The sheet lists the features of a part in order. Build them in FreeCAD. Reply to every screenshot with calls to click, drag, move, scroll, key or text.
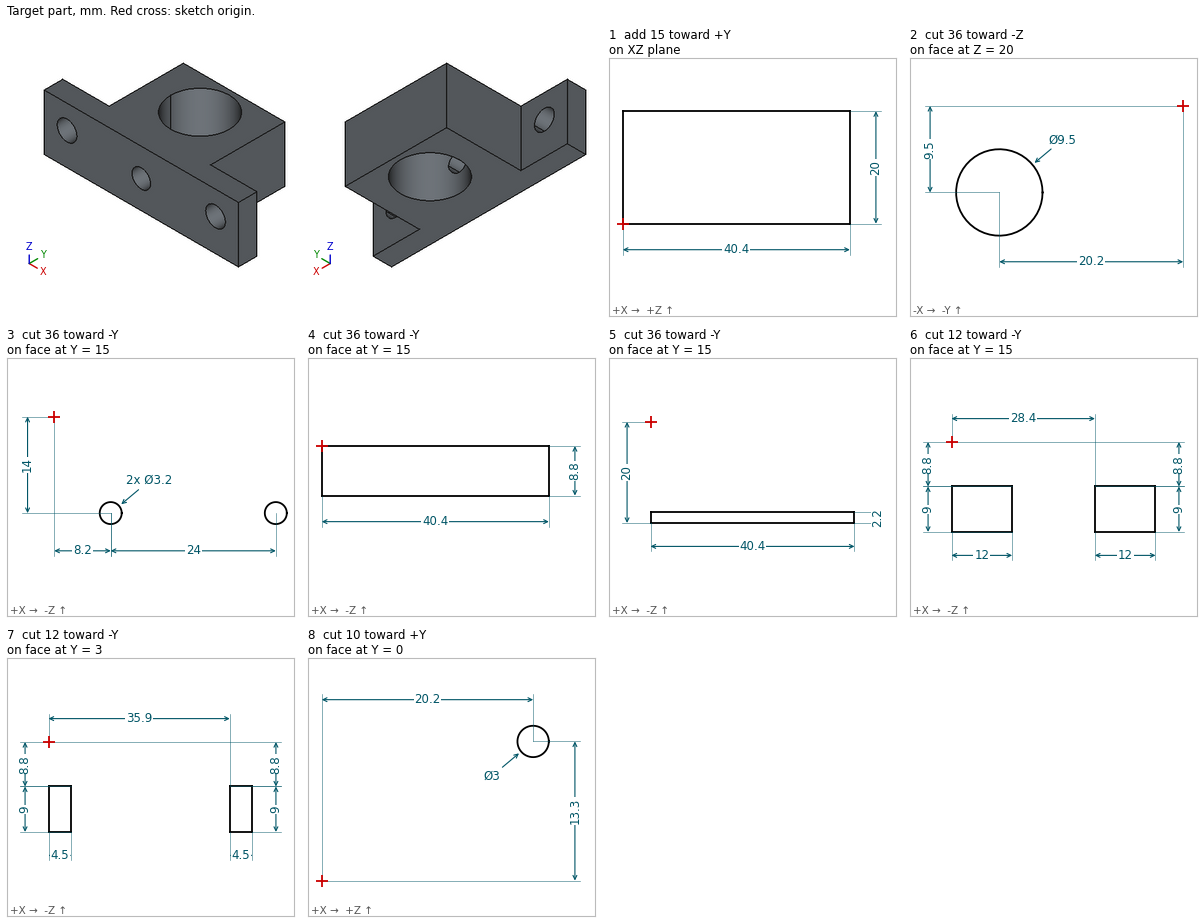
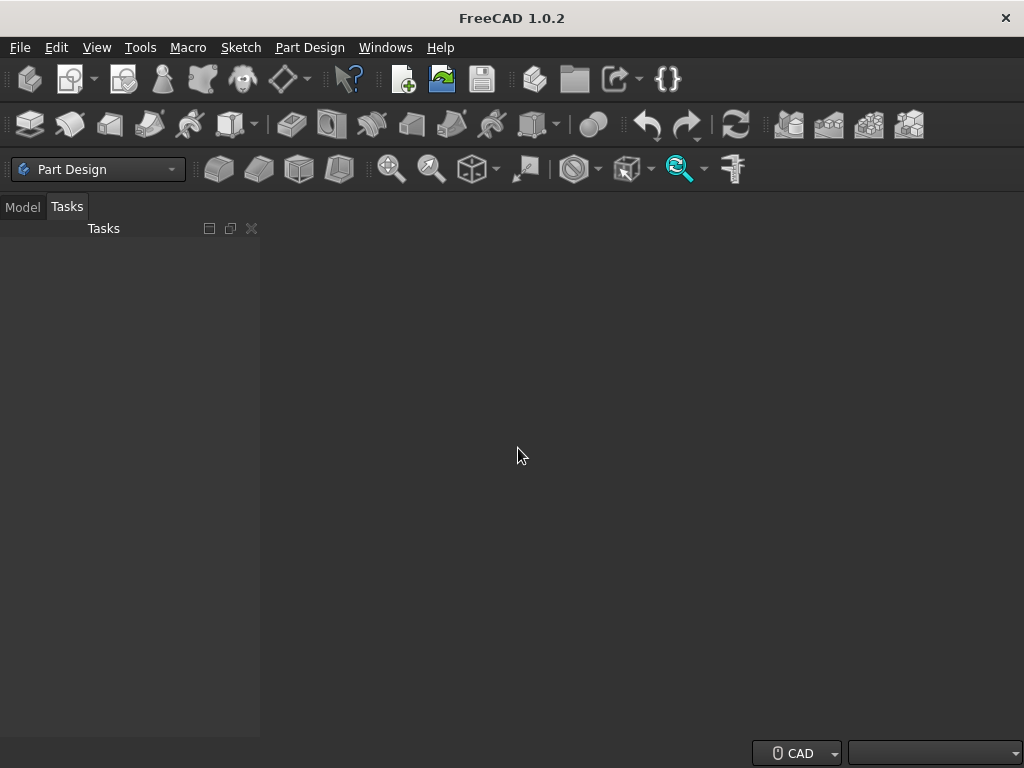
key(ctrl+n)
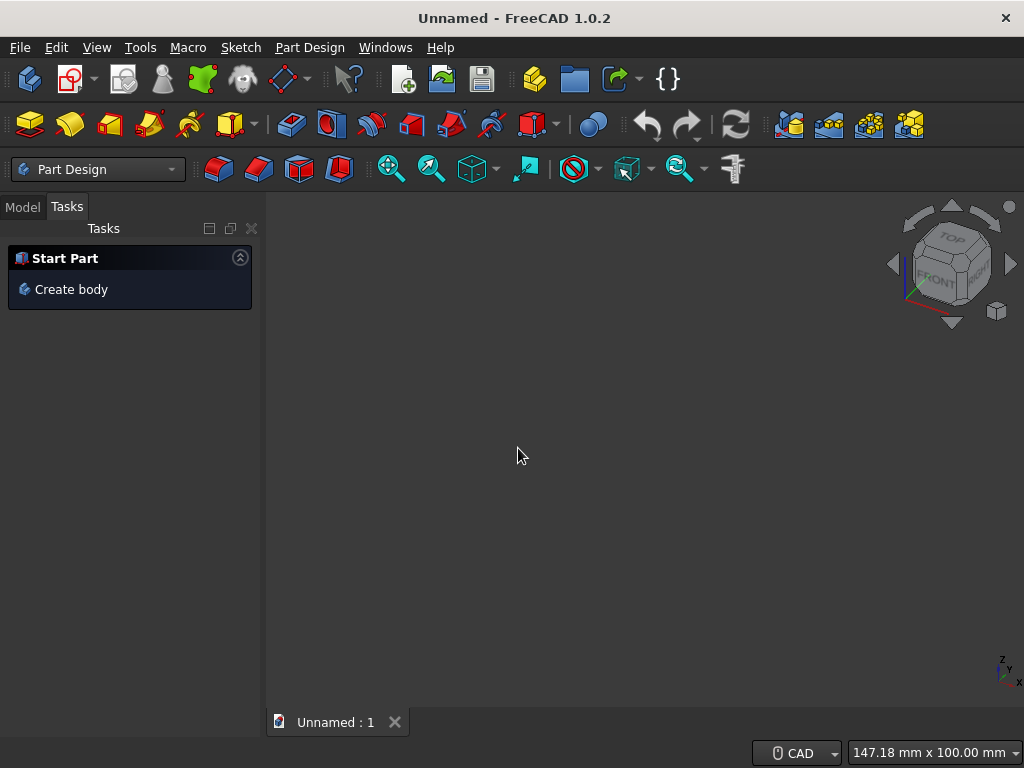
click(70, 80)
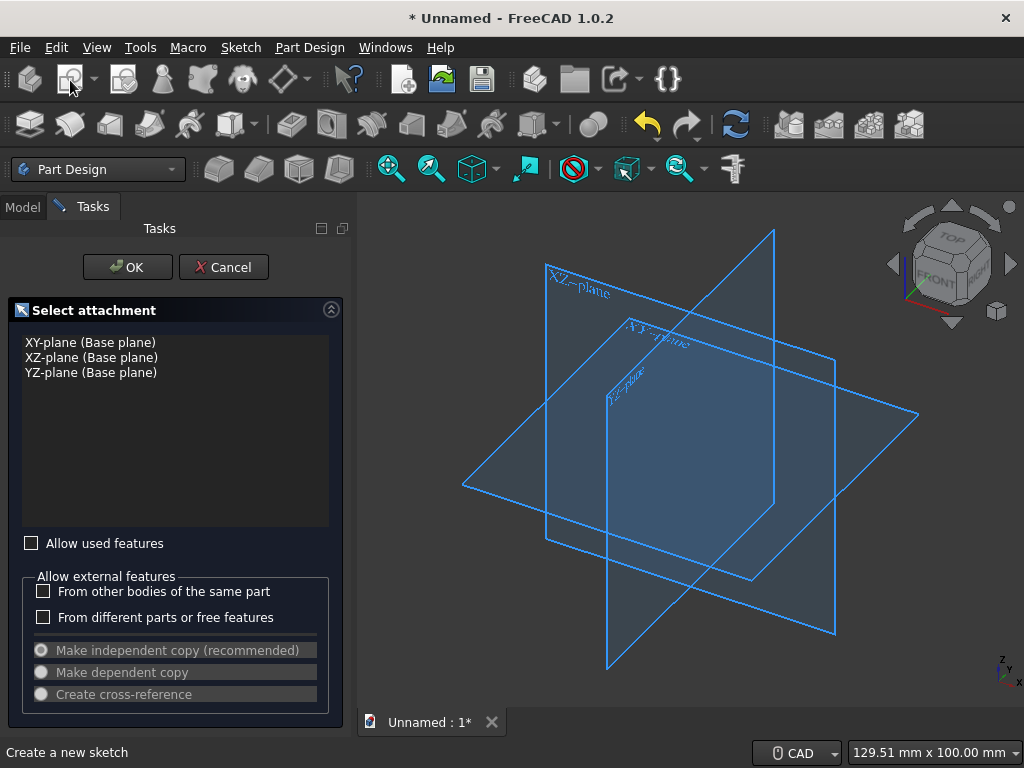
click(82, 358)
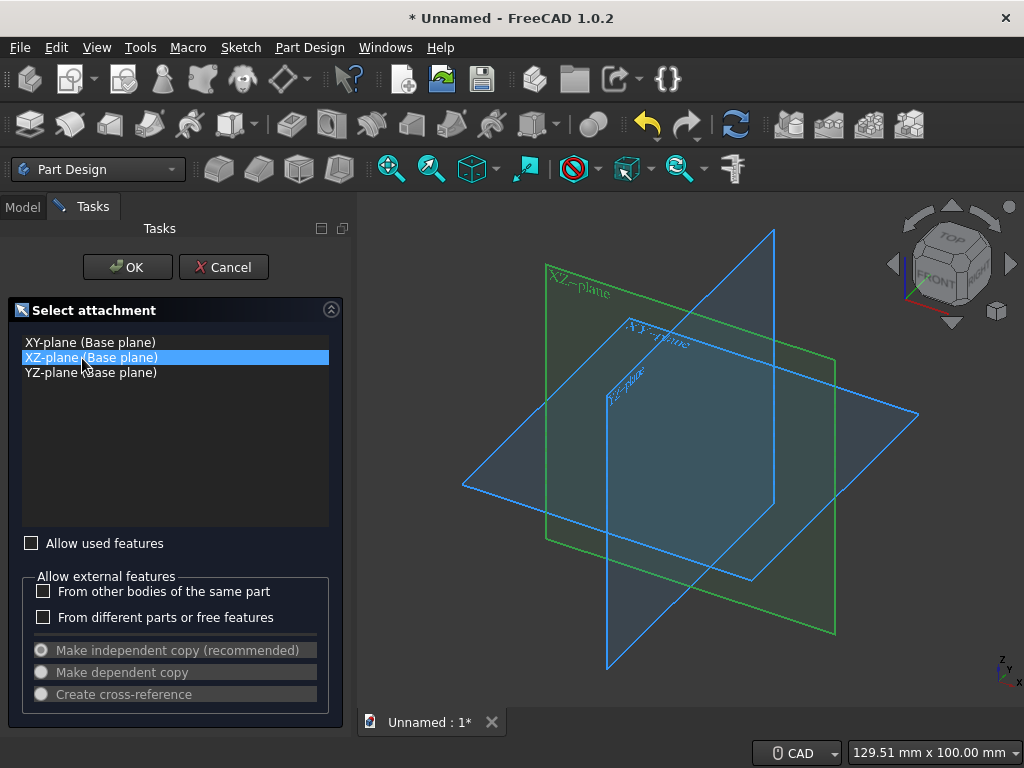
click(128, 267)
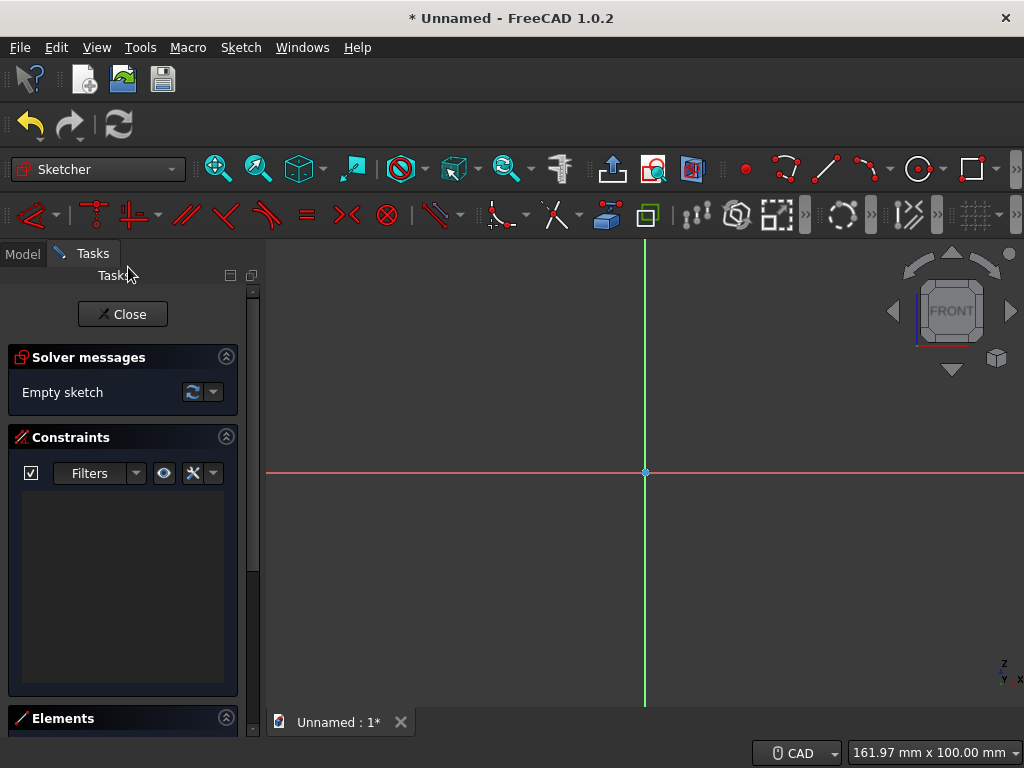
scroll(859, 388, up, 4)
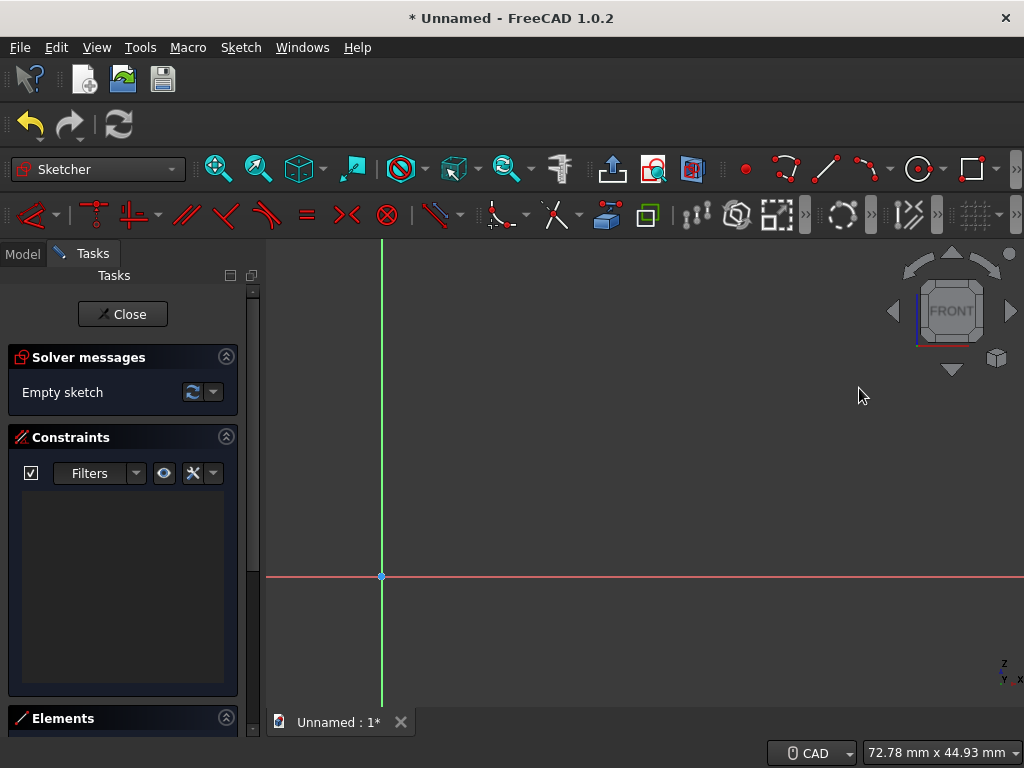
key(g)
key(r)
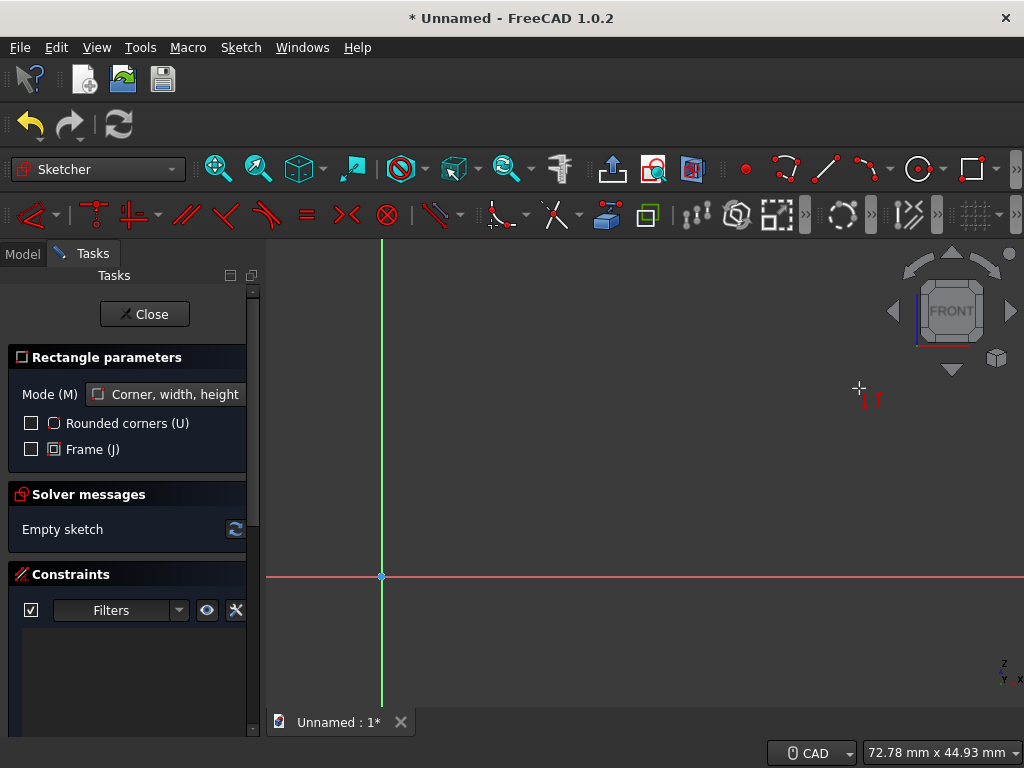
click(382, 577)
move(803, 368)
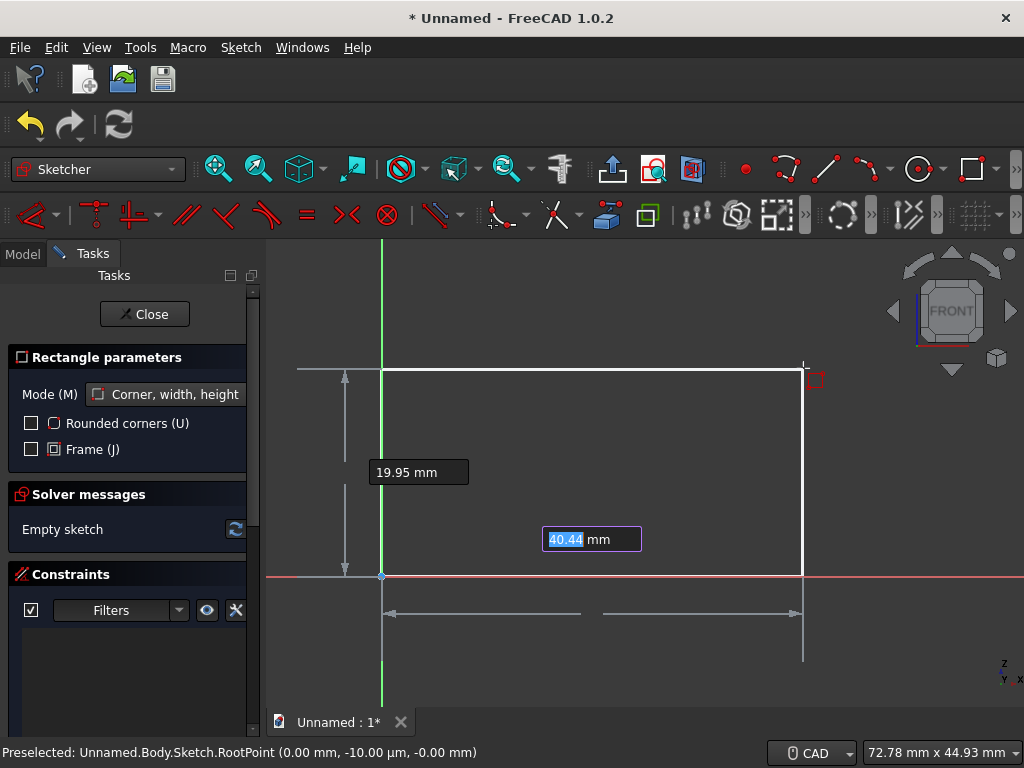
text(40.4)
key(Tab)
text(20)
key(Return)
key(Escape)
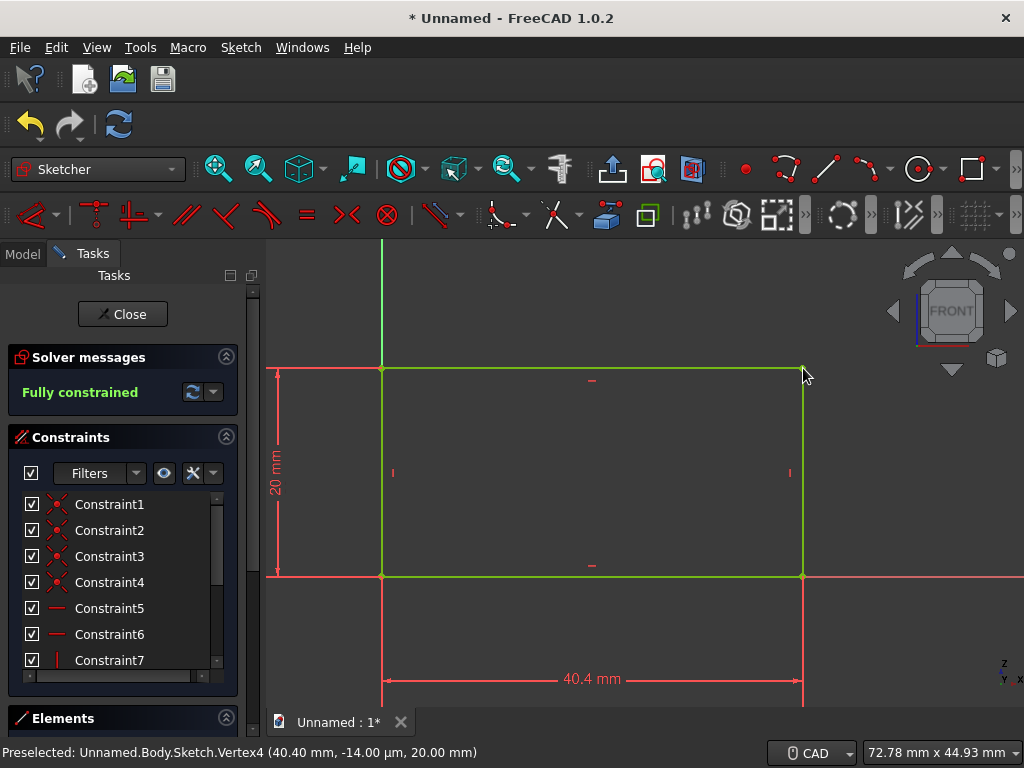
click(123, 314)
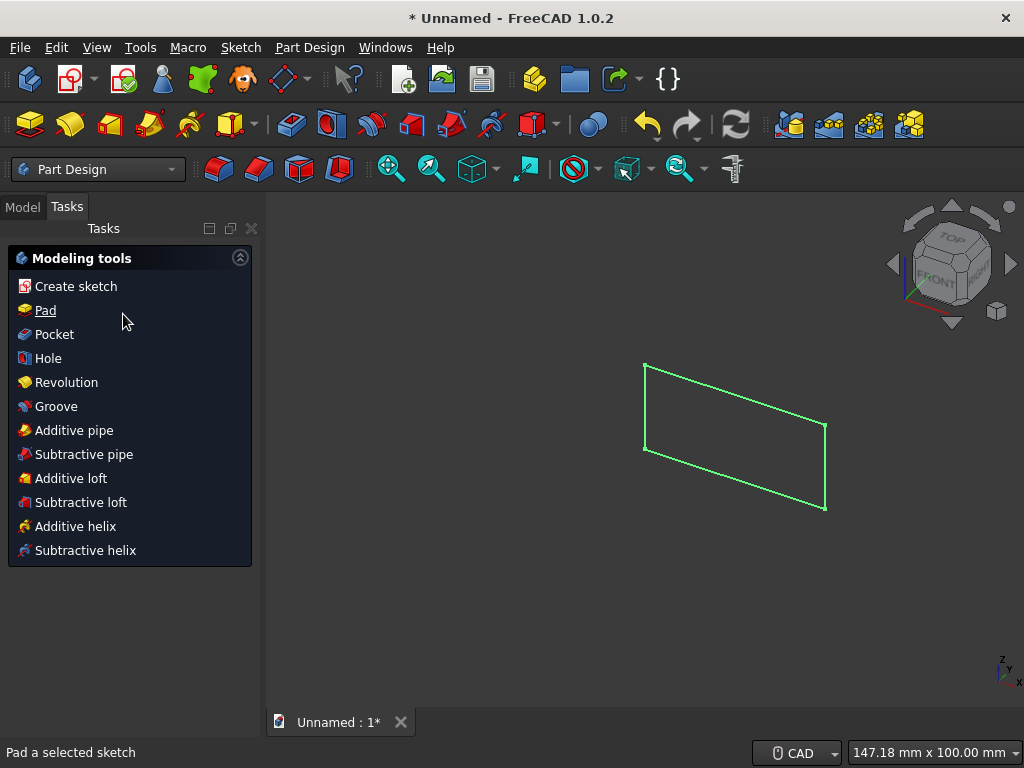
click(30, 124)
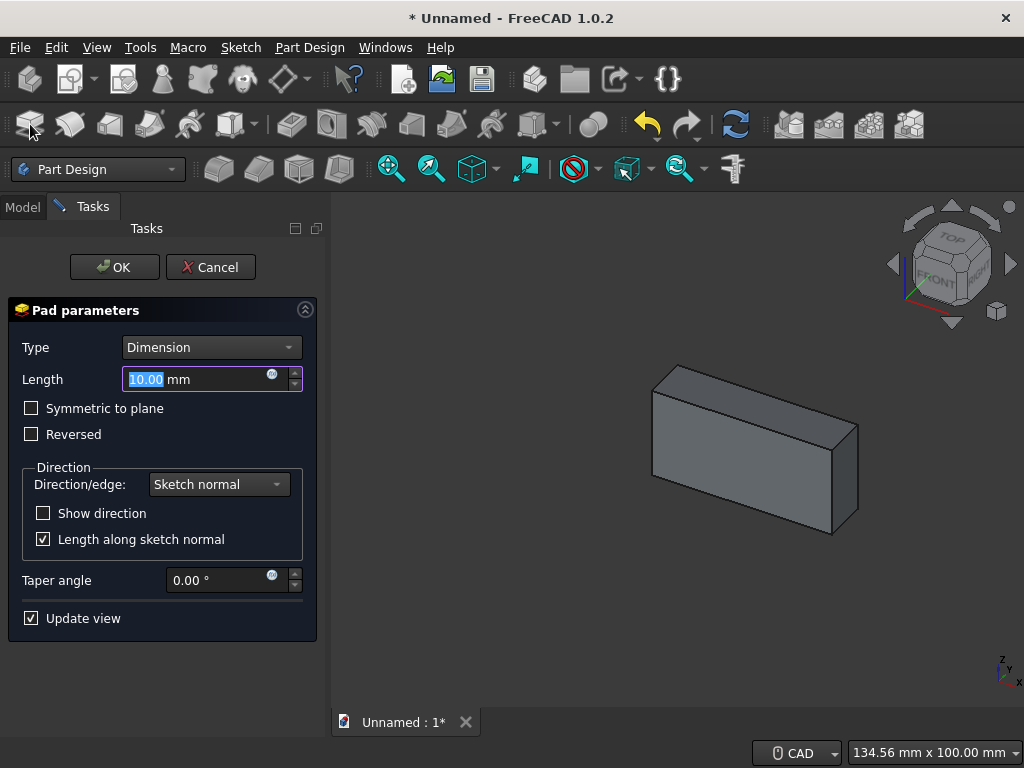
text(15)
key(Tab)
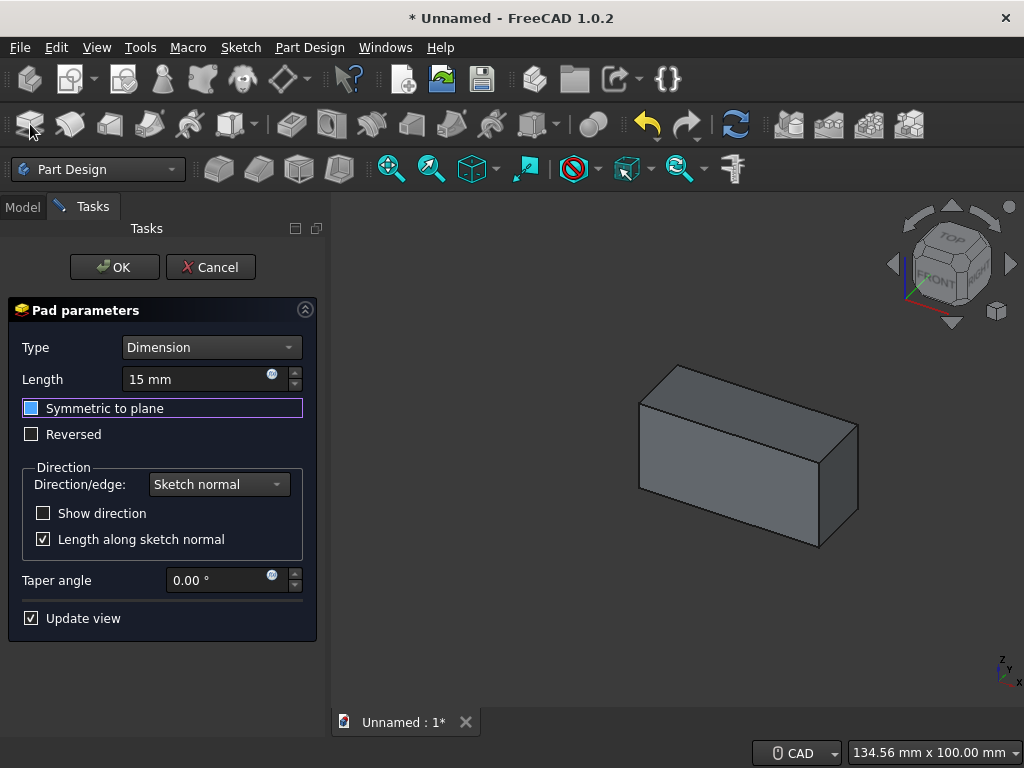
click(30, 434)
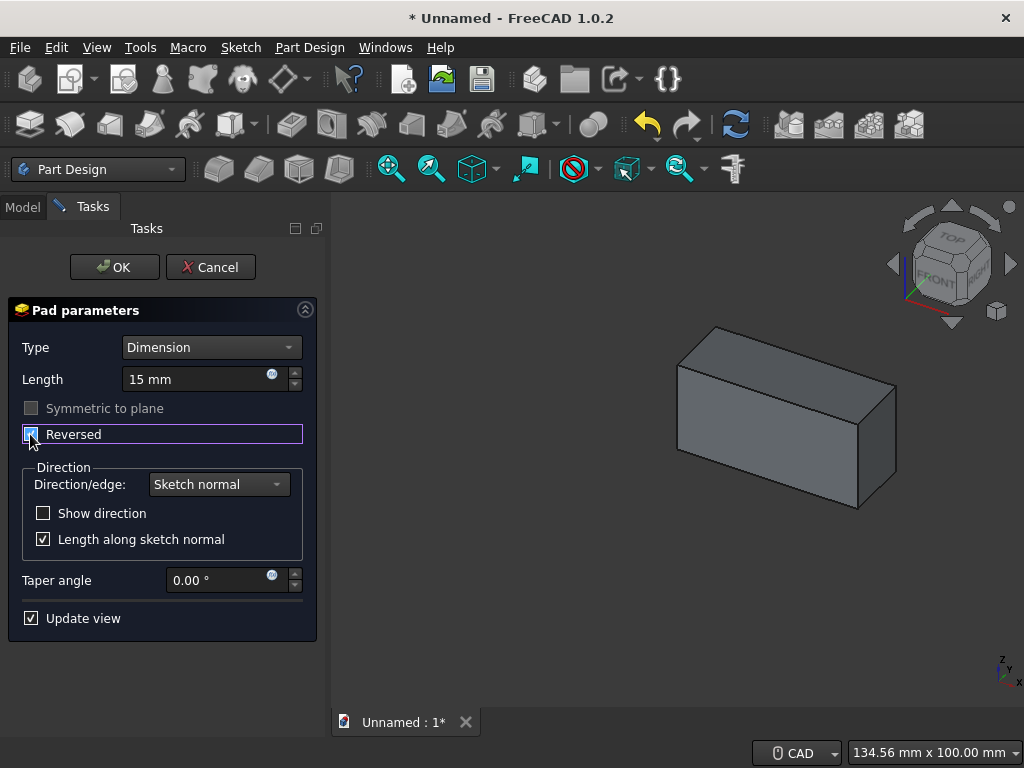
click(115, 267)